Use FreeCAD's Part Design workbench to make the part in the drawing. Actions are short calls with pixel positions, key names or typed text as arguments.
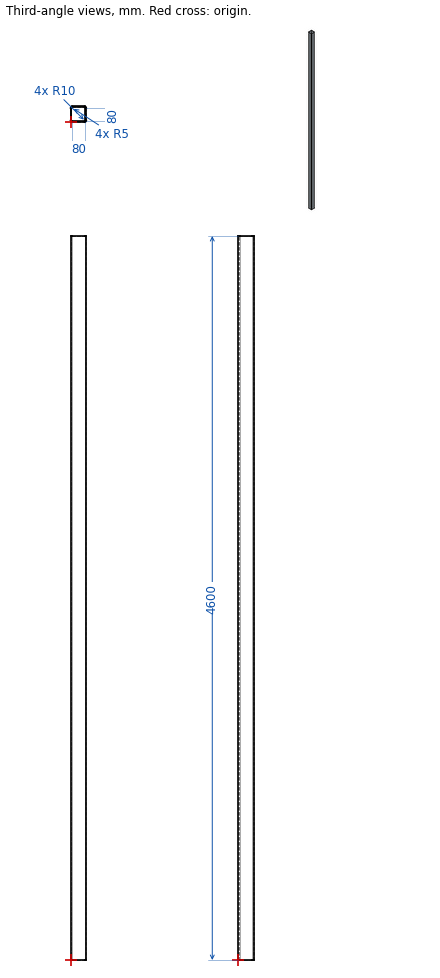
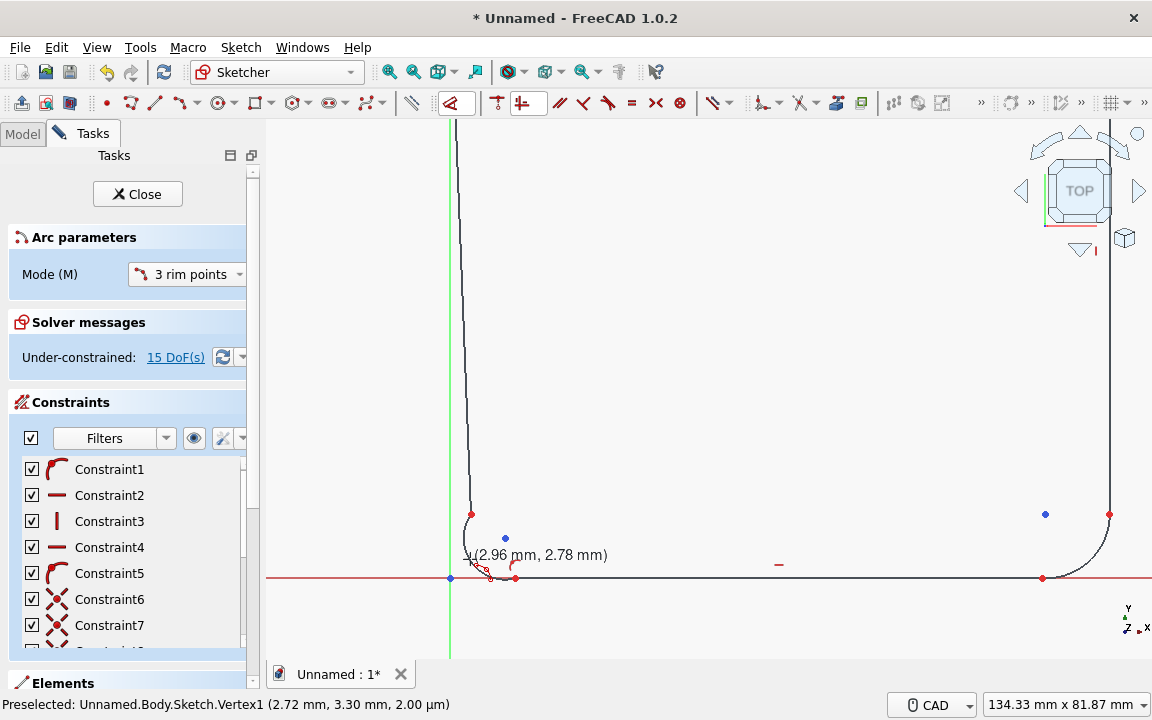
key(g)
key(l)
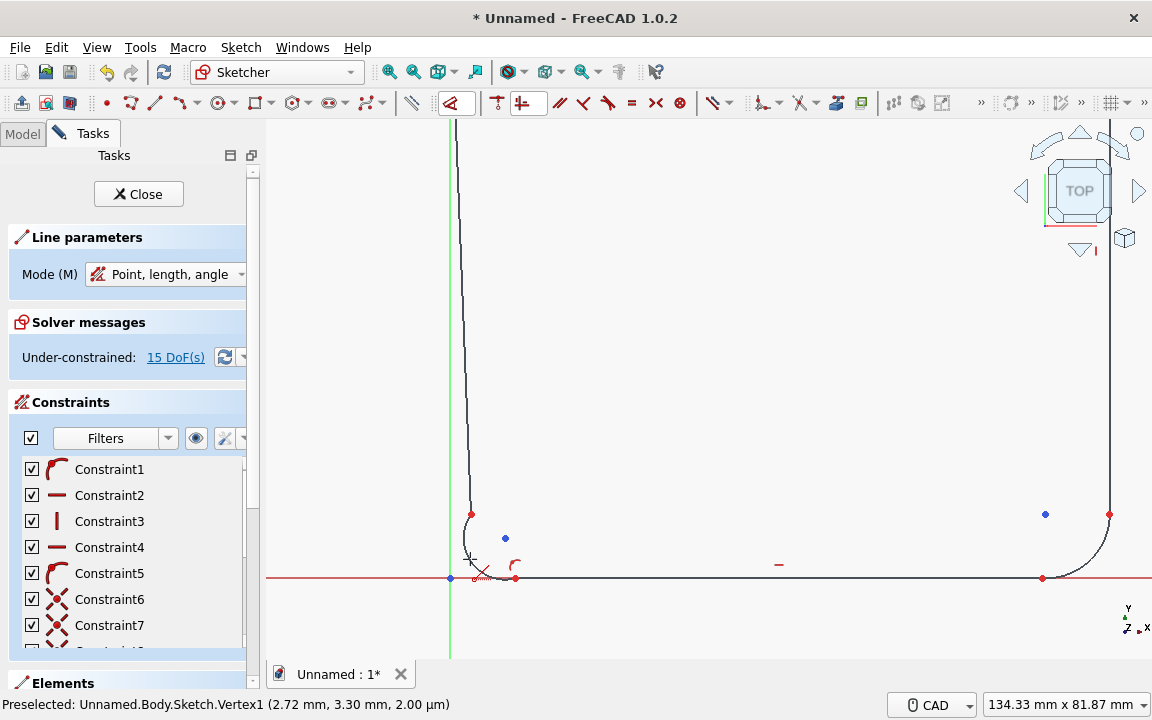
scroll(470, 560, down, 3)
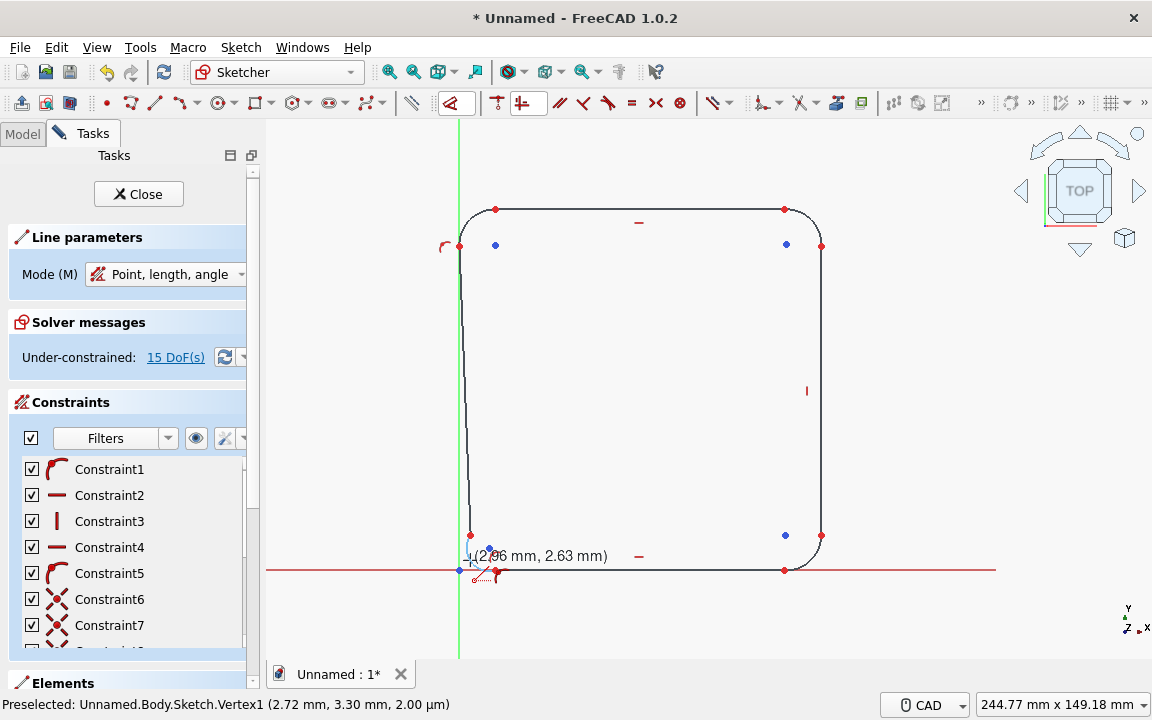
click(496, 227)
click(785, 227)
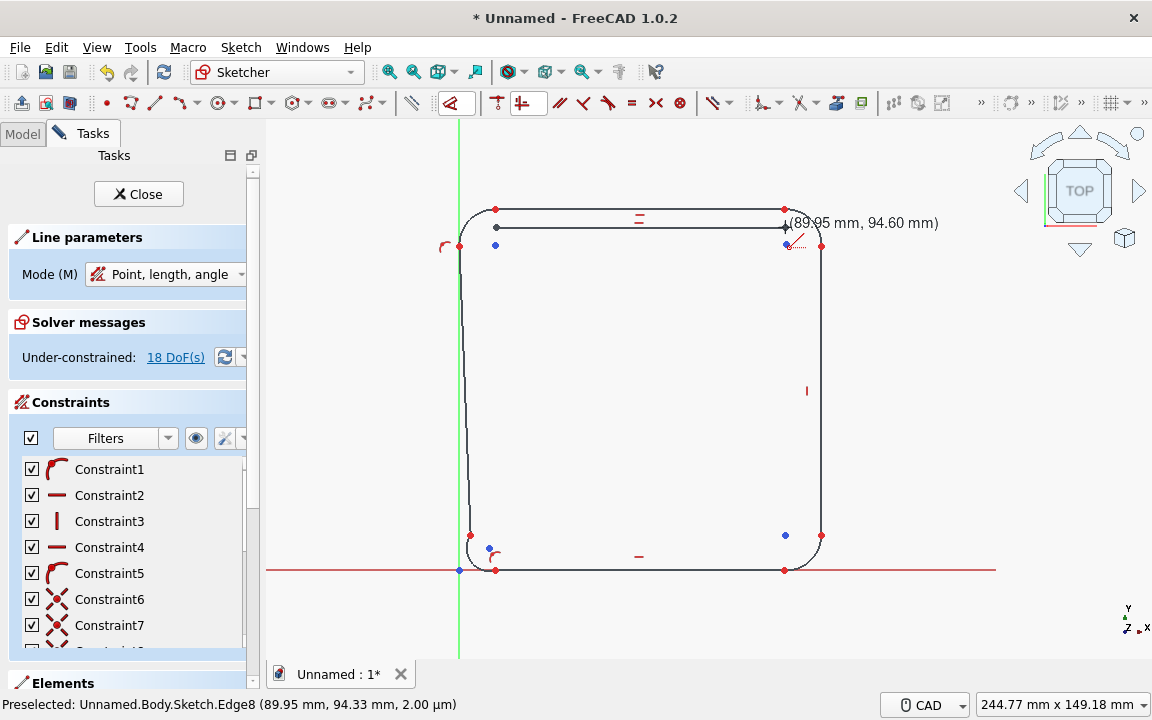
click(803, 245)
click(803, 534)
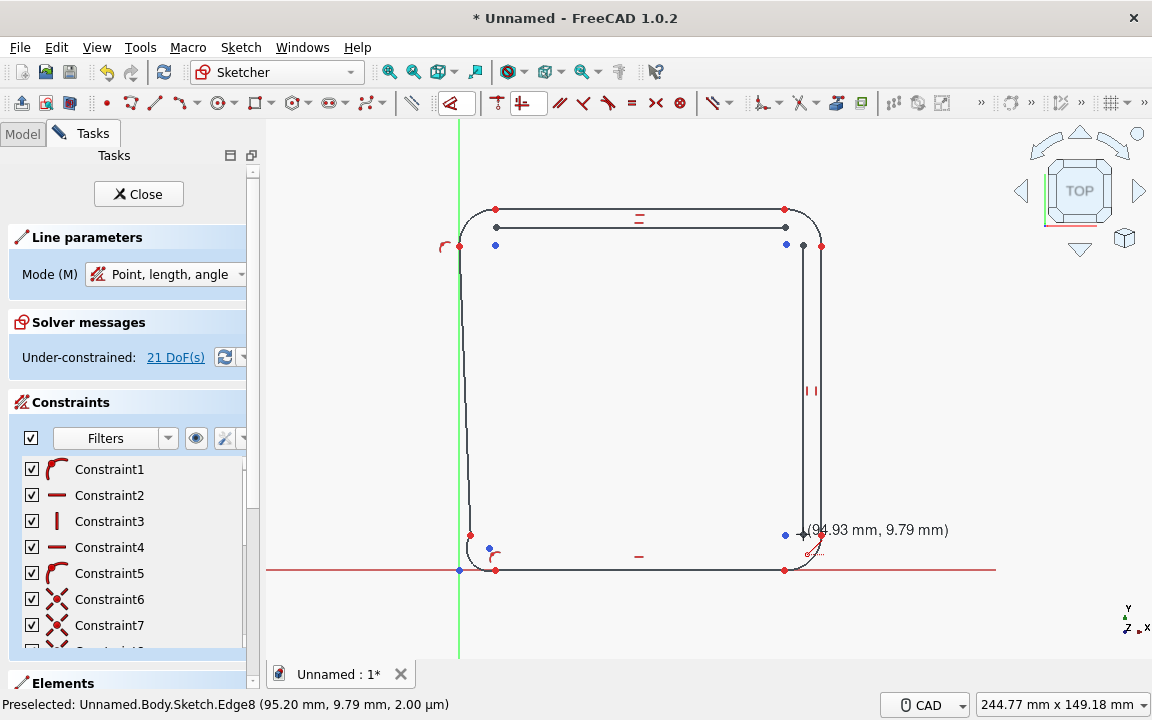
click(785, 552)
click(496, 552)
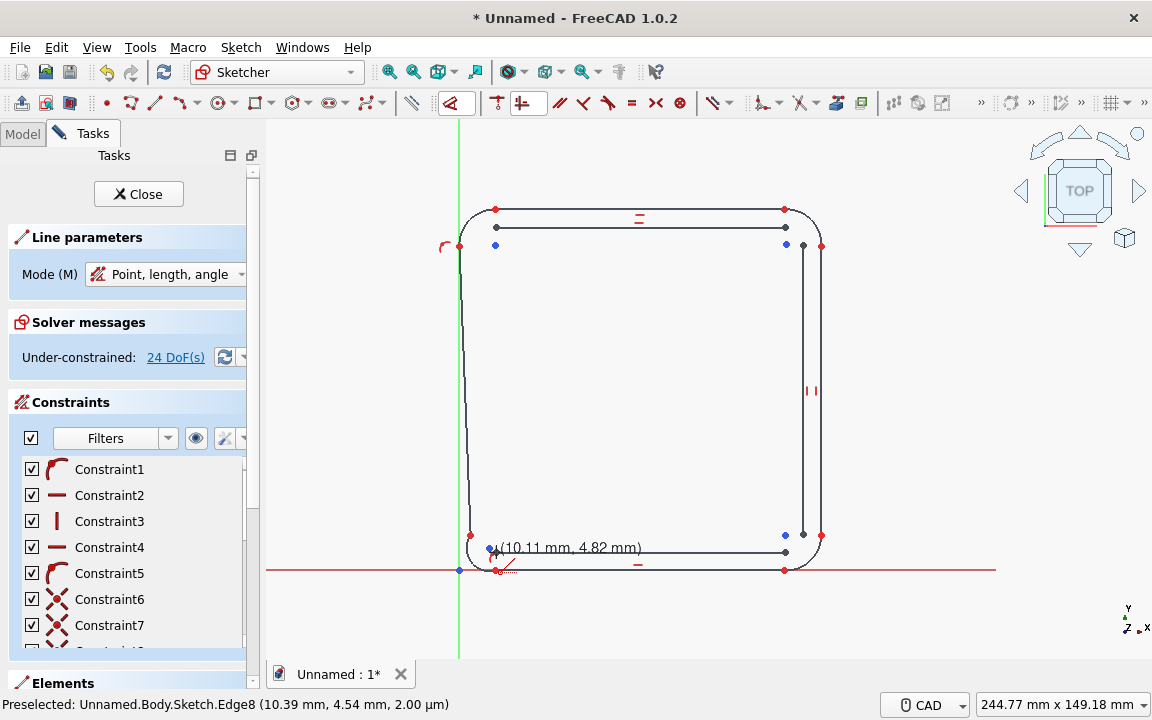
click(477, 534)
click(477, 245)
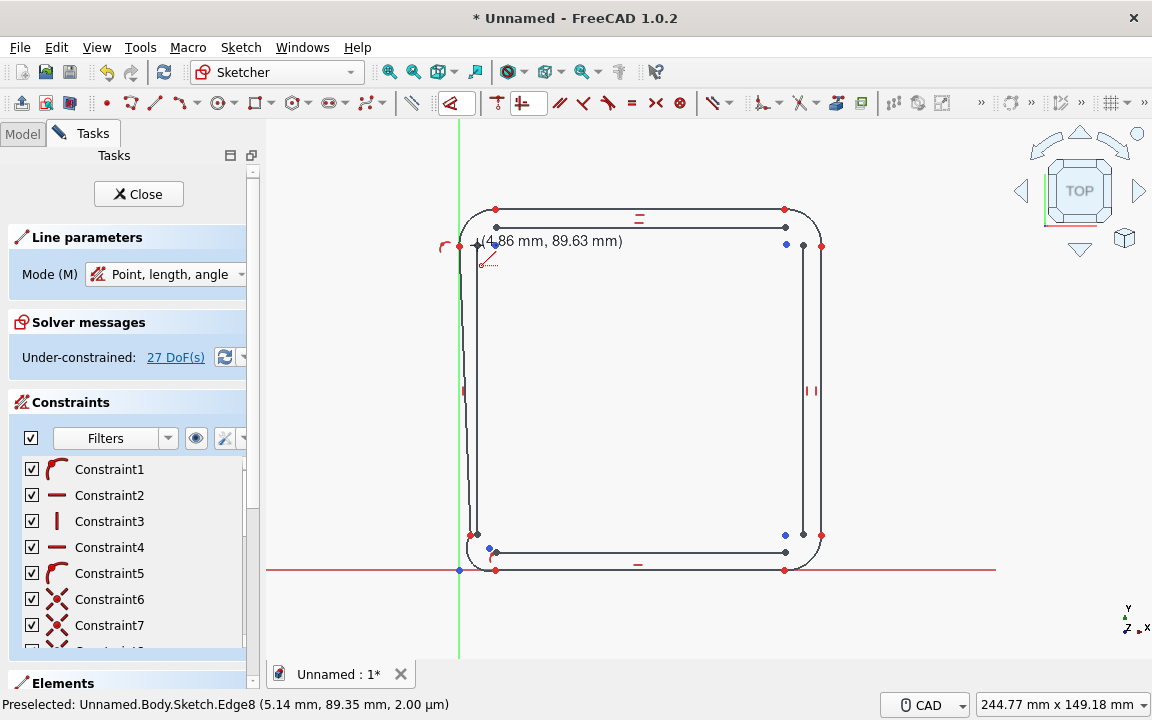
click(180, 104)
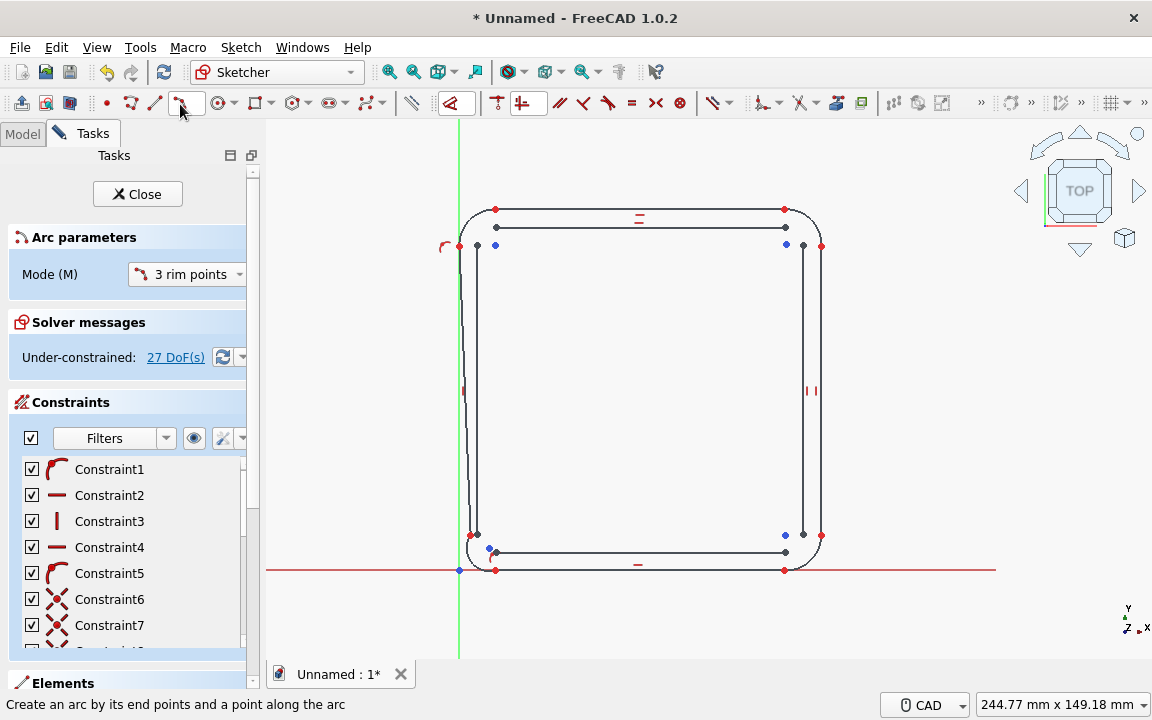
click(785, 228)
click(803, 246)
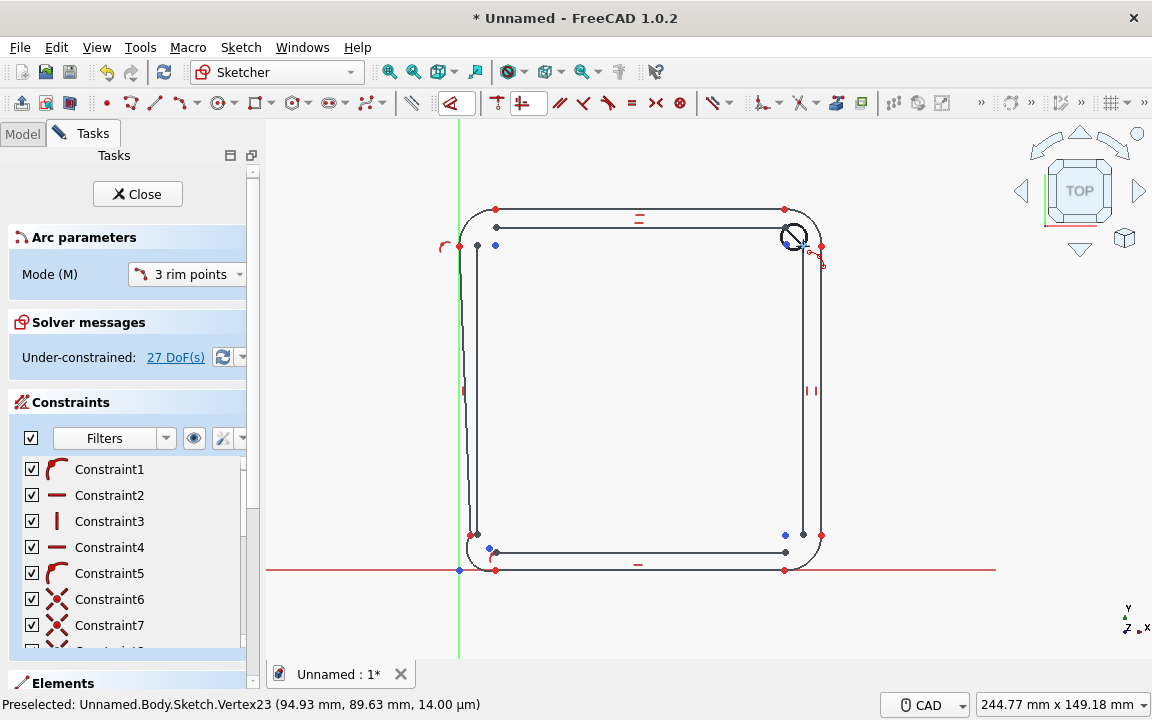
scroll(798, 232, up, 6)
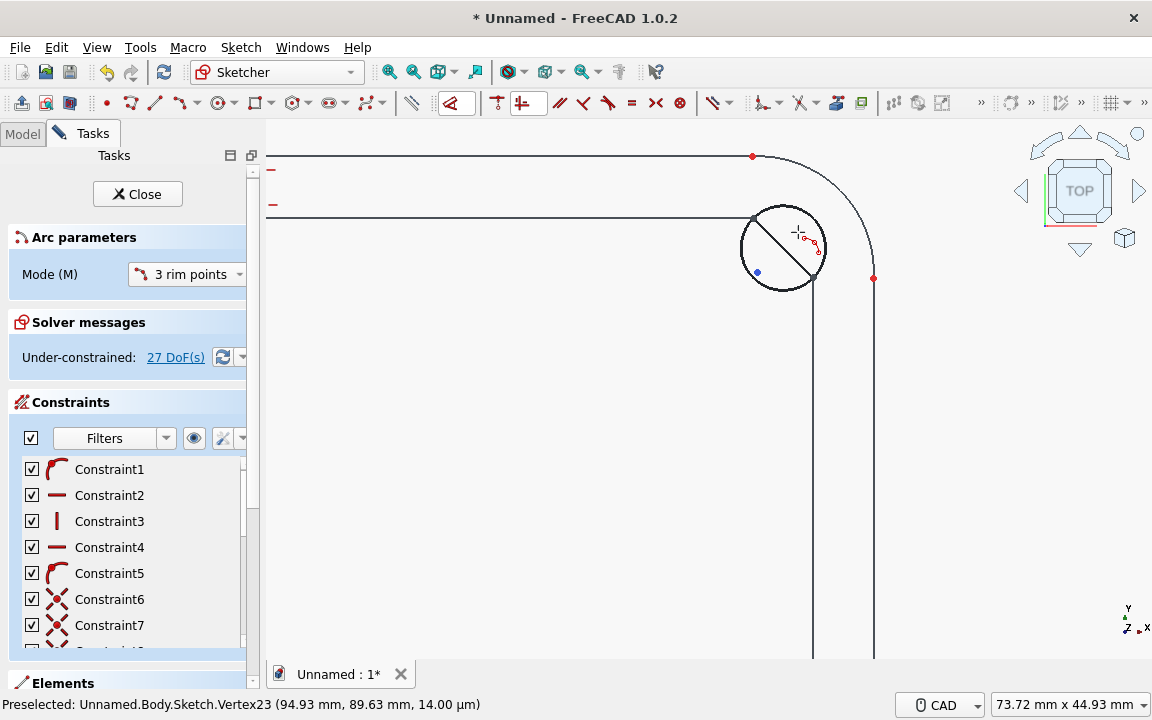
click(797, 231)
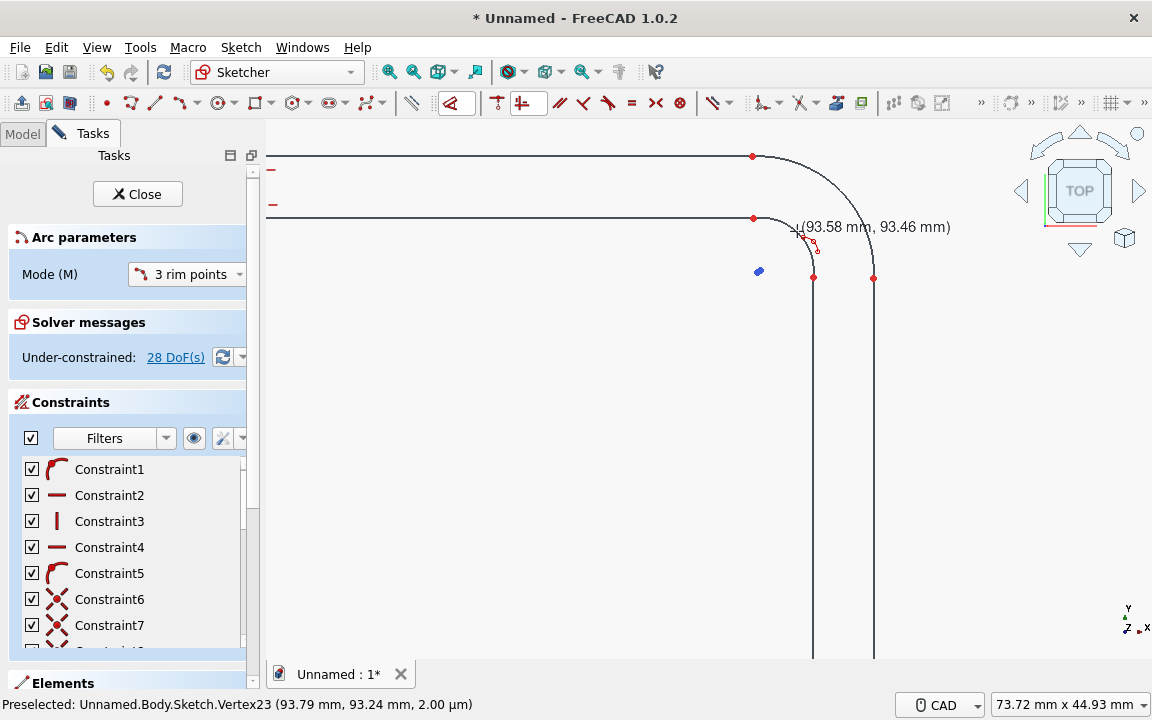
scroll(799, 232, down, 6)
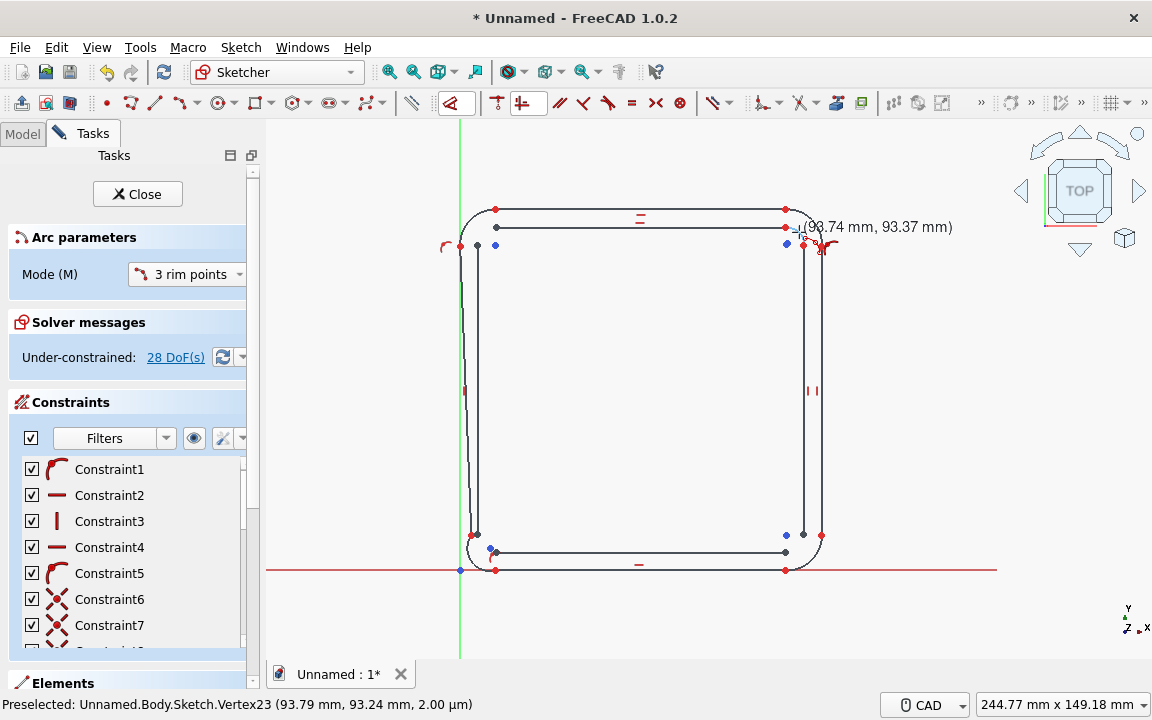
click(804, 535)
click(786, 553)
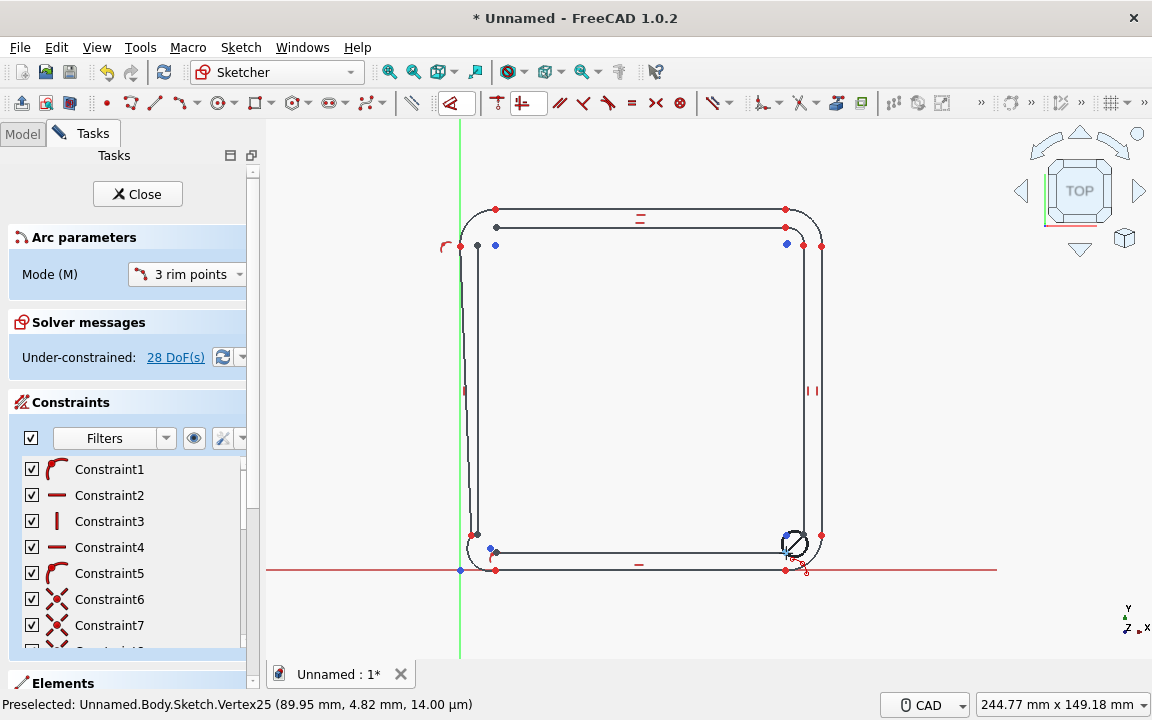
scroll(799, 547, up, 6)